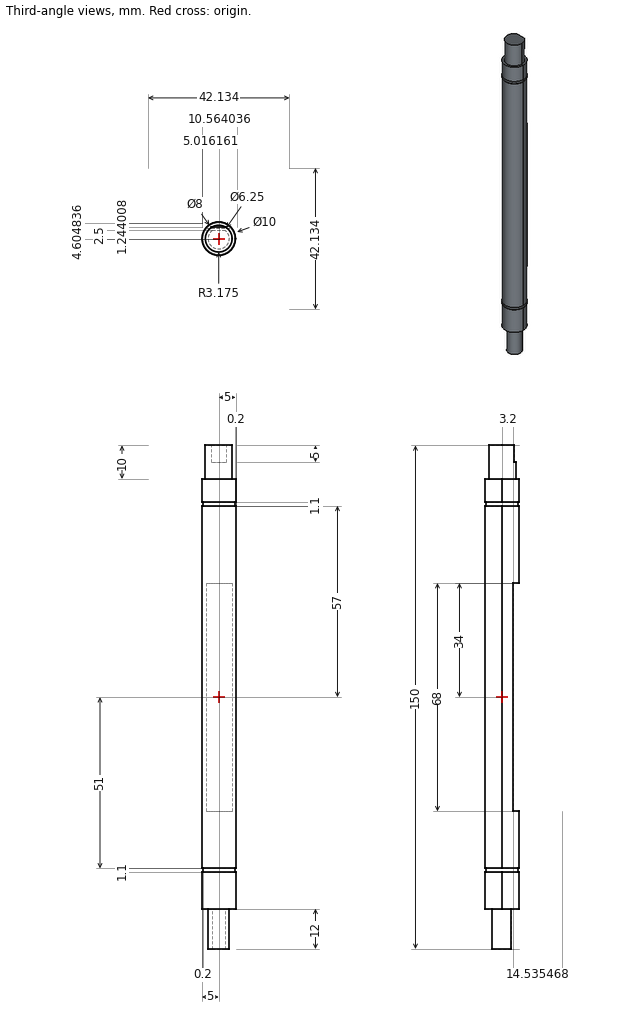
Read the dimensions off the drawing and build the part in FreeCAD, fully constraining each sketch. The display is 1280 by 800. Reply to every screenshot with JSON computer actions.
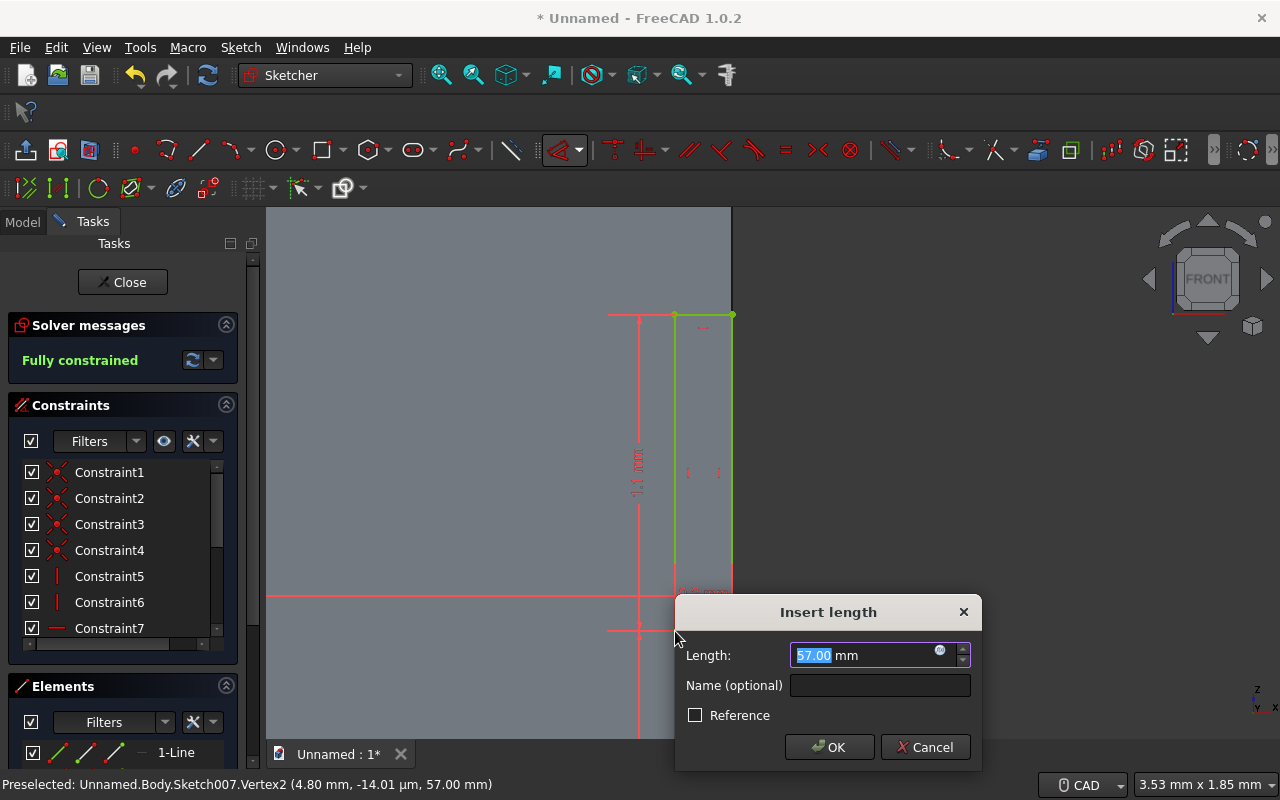
{"action": "type", "text": "57"}
{"action": "key", "text": "Return"}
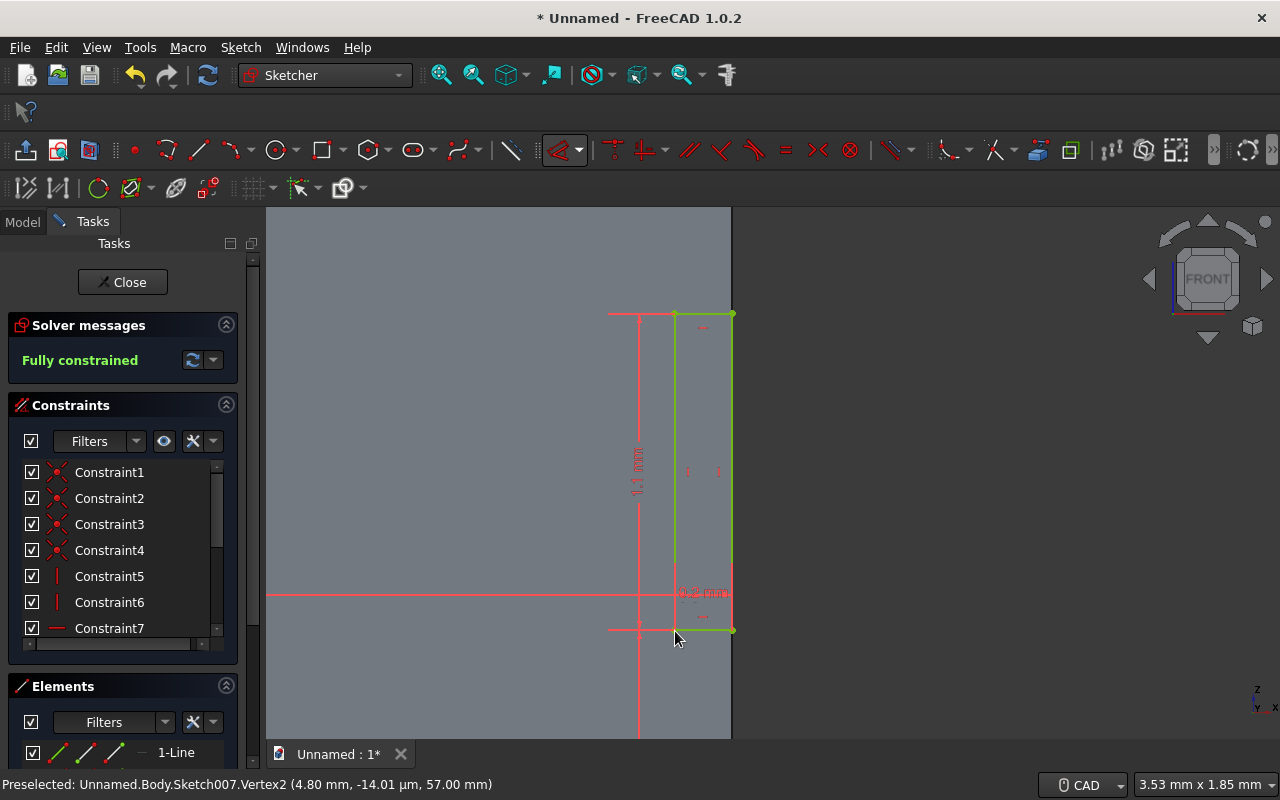
{"action": "left_click", "coordinate": [123, 282]}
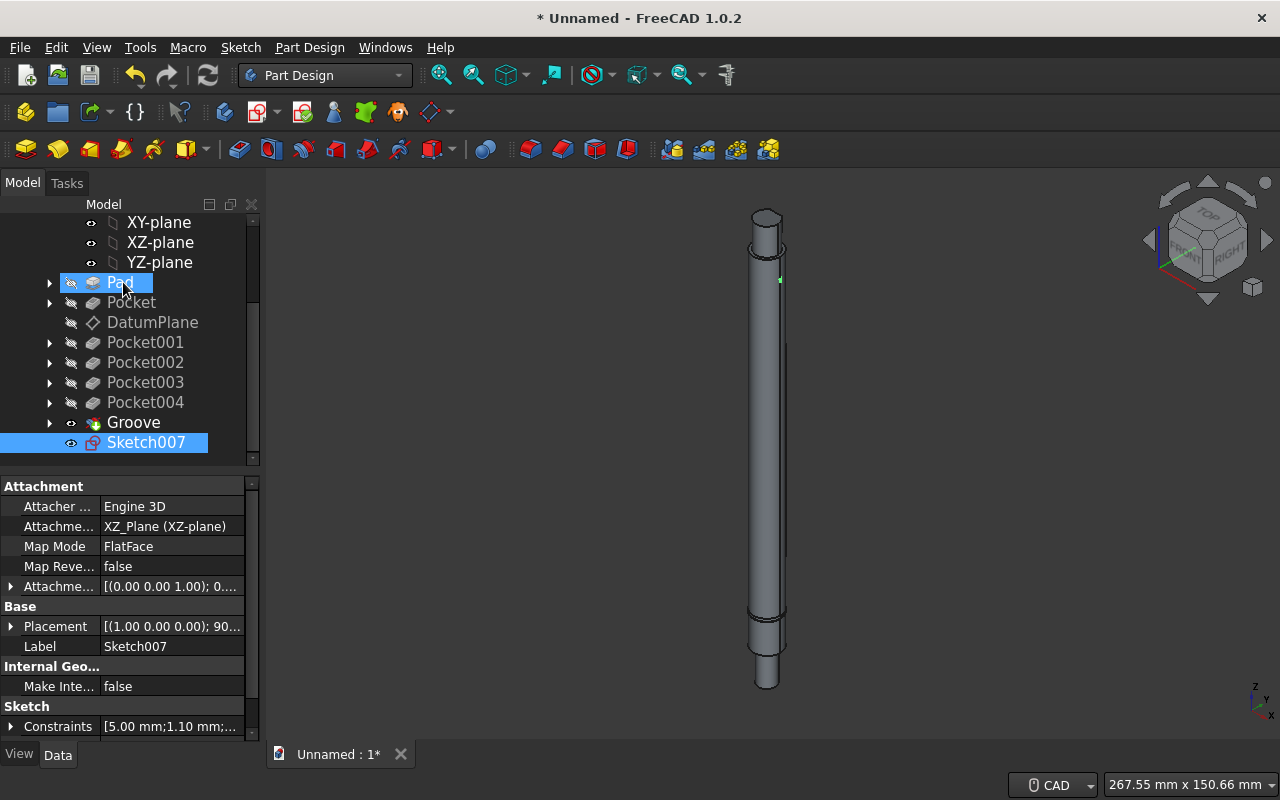
{"action": "left_click", "coordinate": [304, 150]}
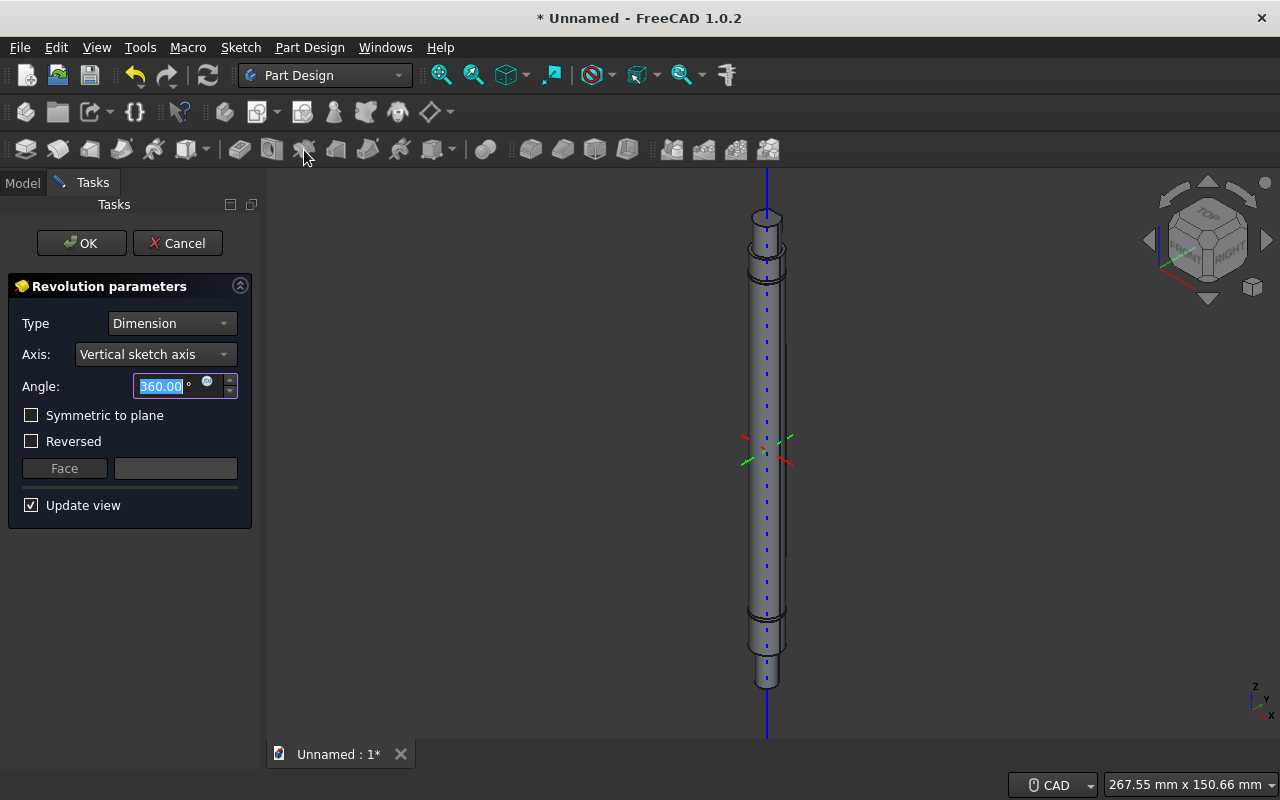
{"action": "left_click", "coordinate": [82, 243]}